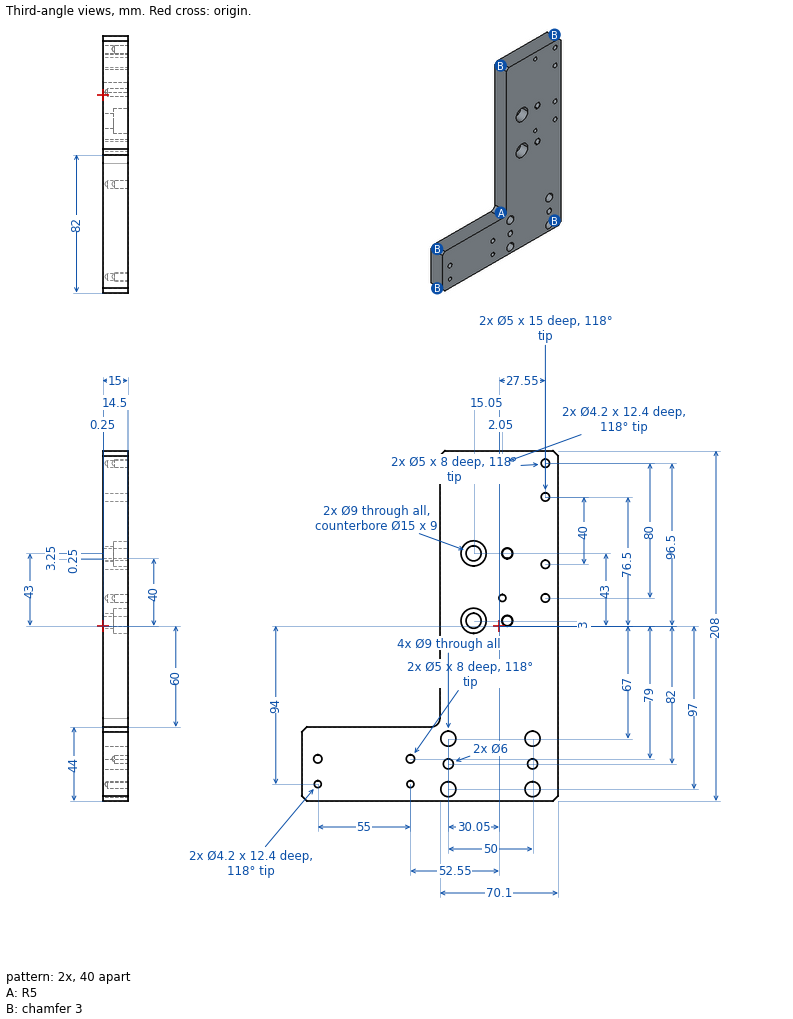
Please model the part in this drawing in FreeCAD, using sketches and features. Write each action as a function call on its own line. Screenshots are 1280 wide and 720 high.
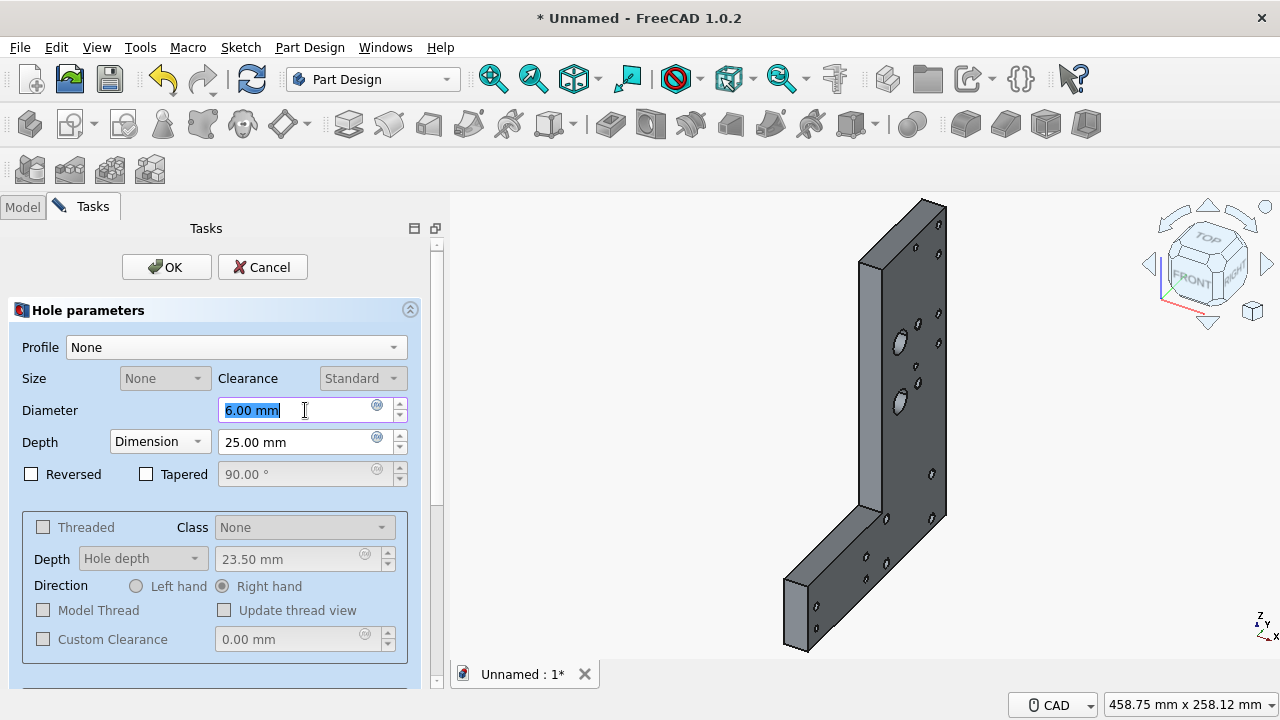
text(9)
key(Tab)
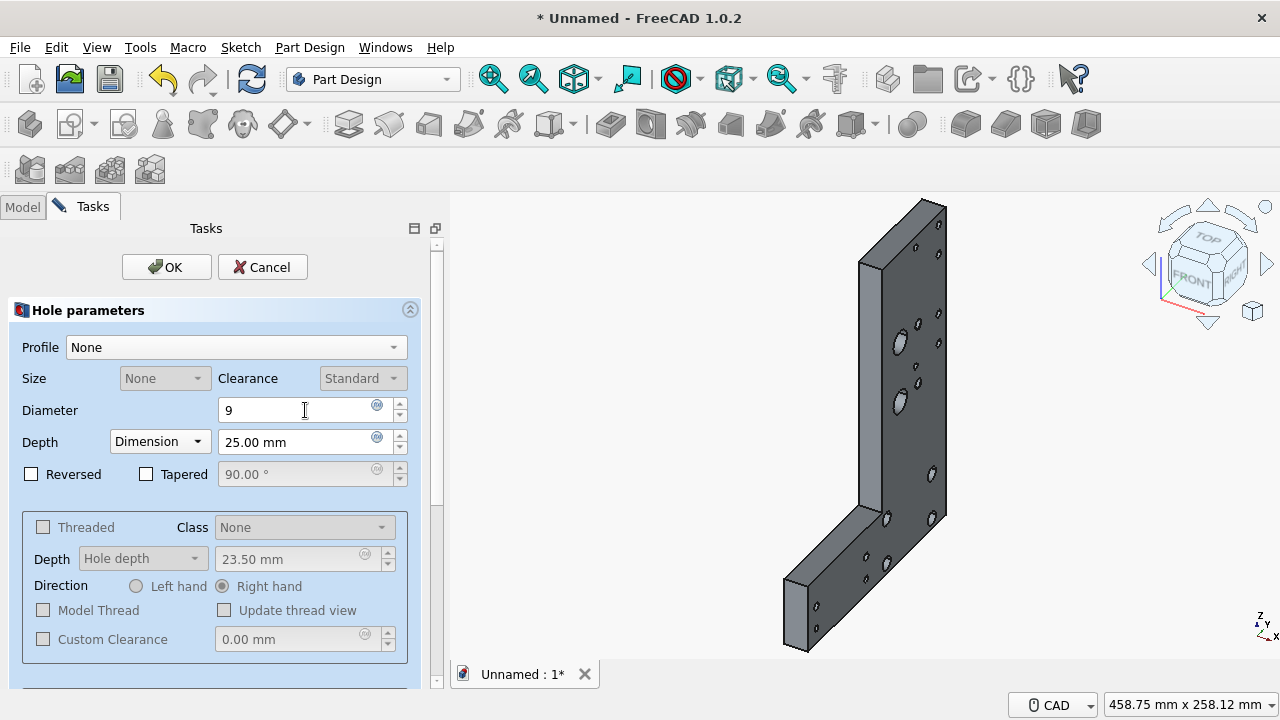
click(161, 442)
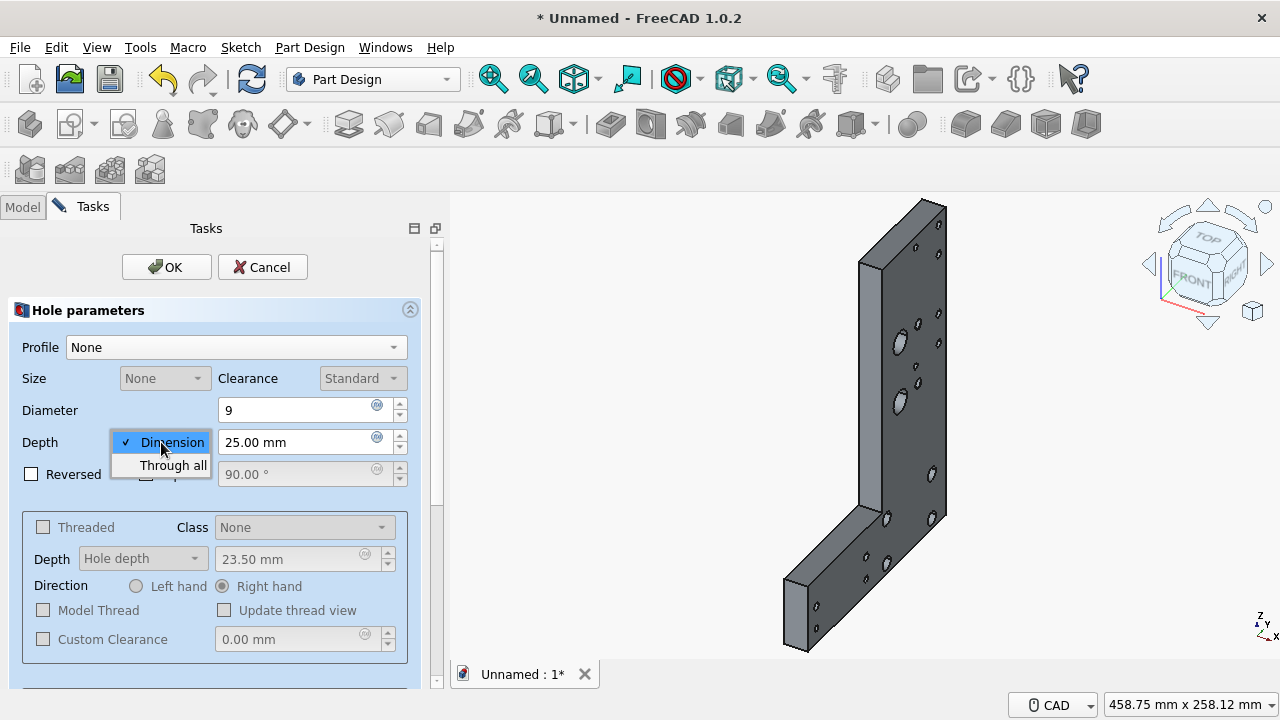
click(160, 466)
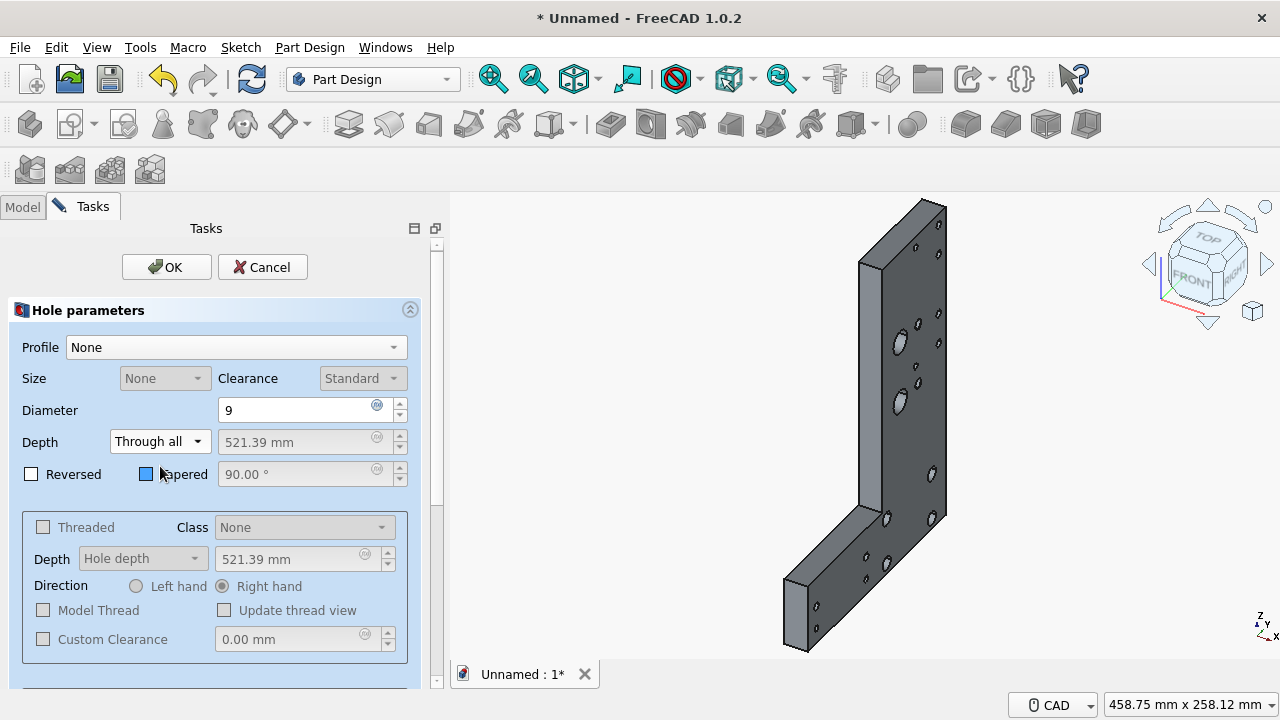
click(167, 267)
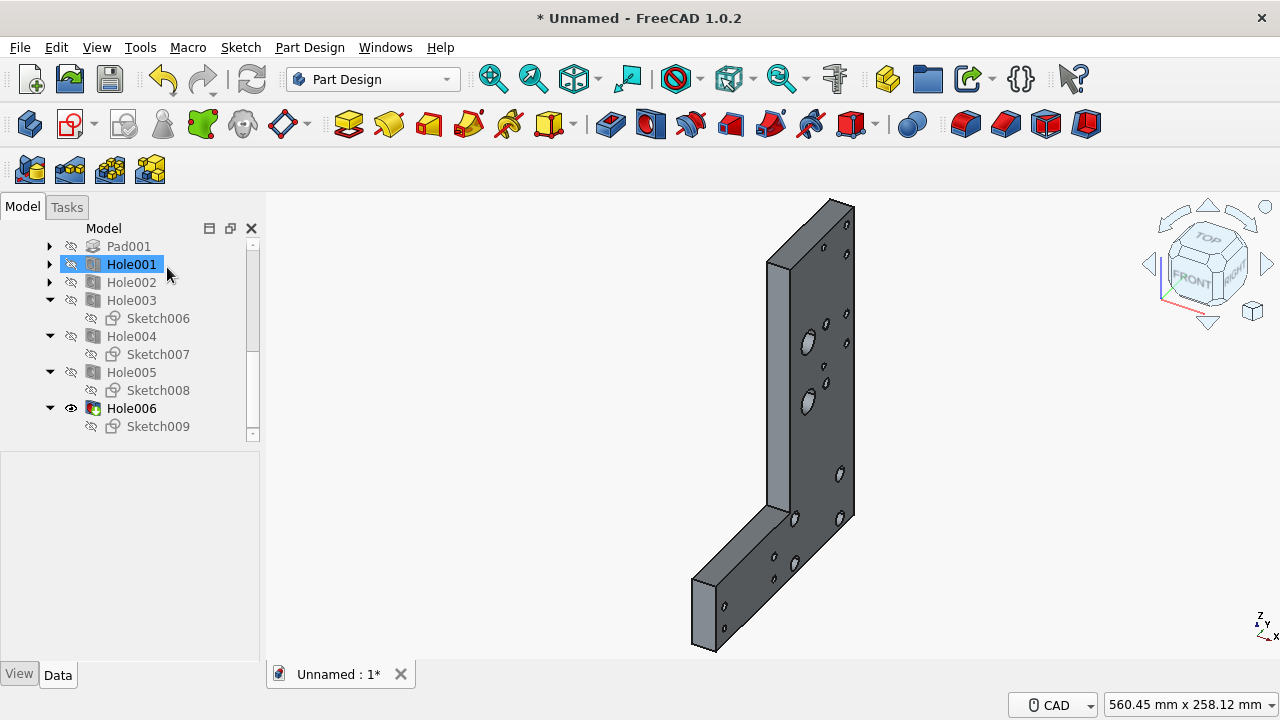
click(824, 433)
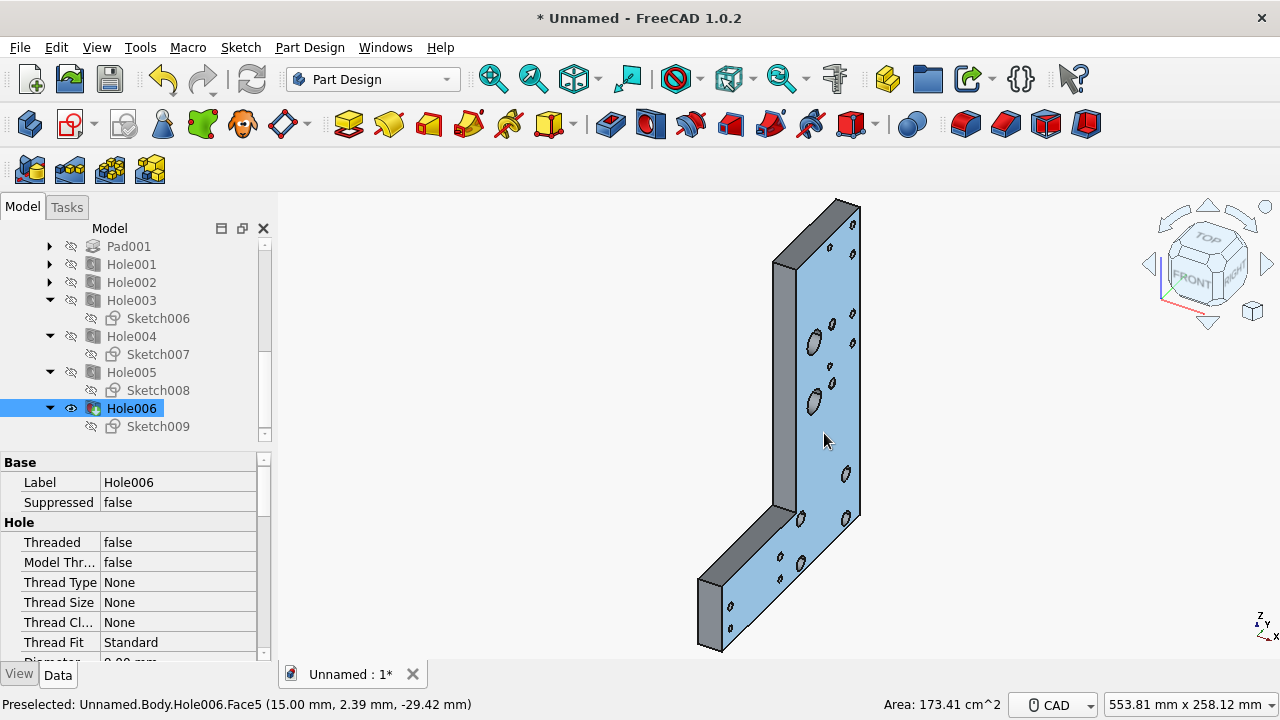
click(70, 124)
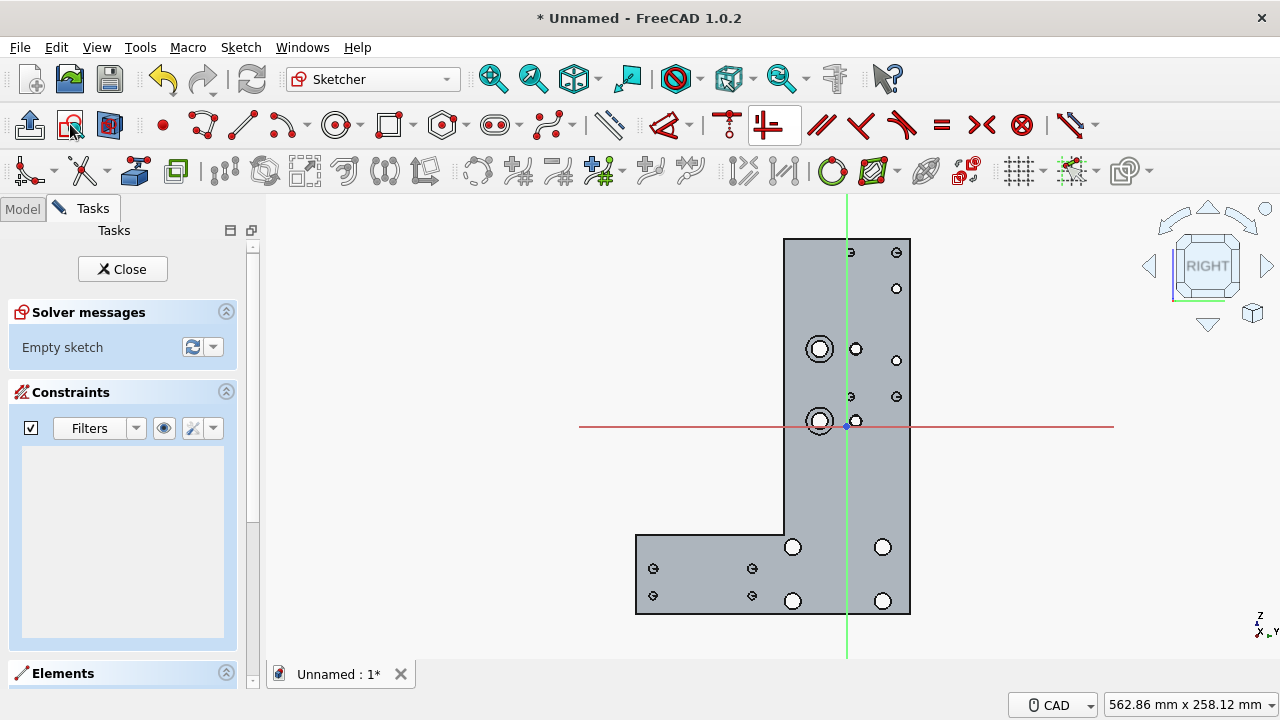
scroll(1000, 596, up, 3)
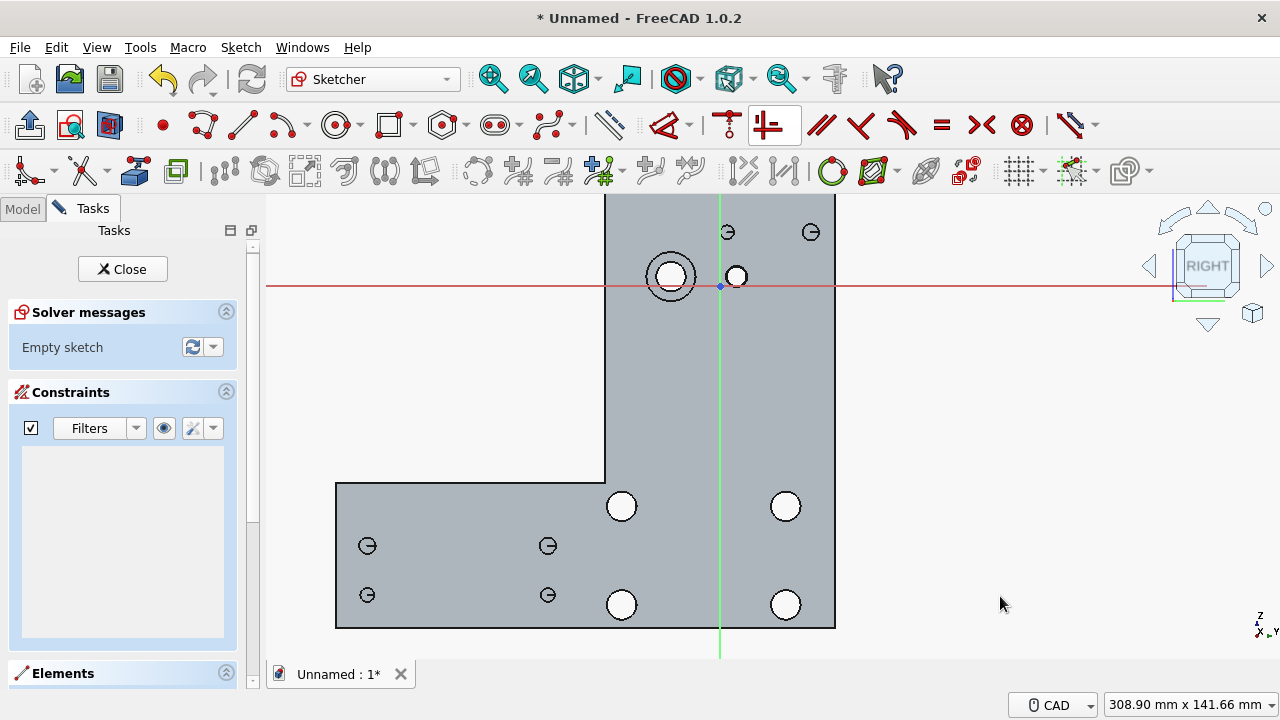
click(336, 126)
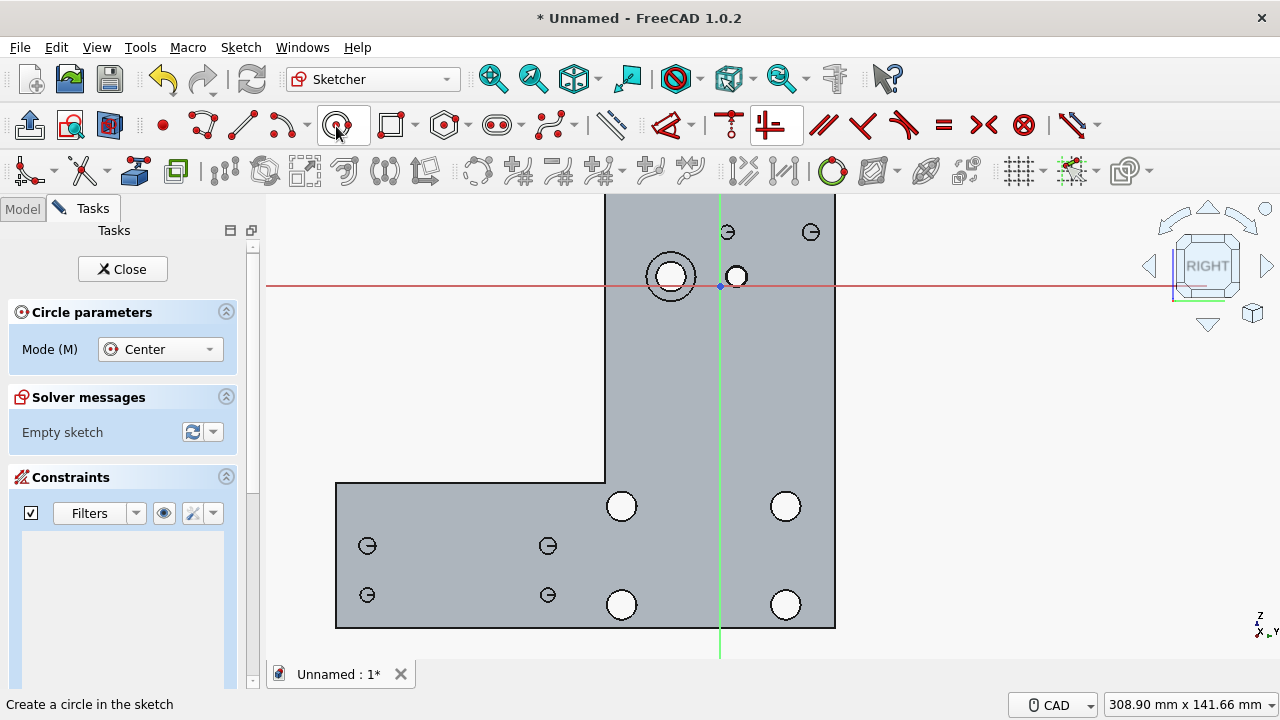
scroll(622, 556, up, 5)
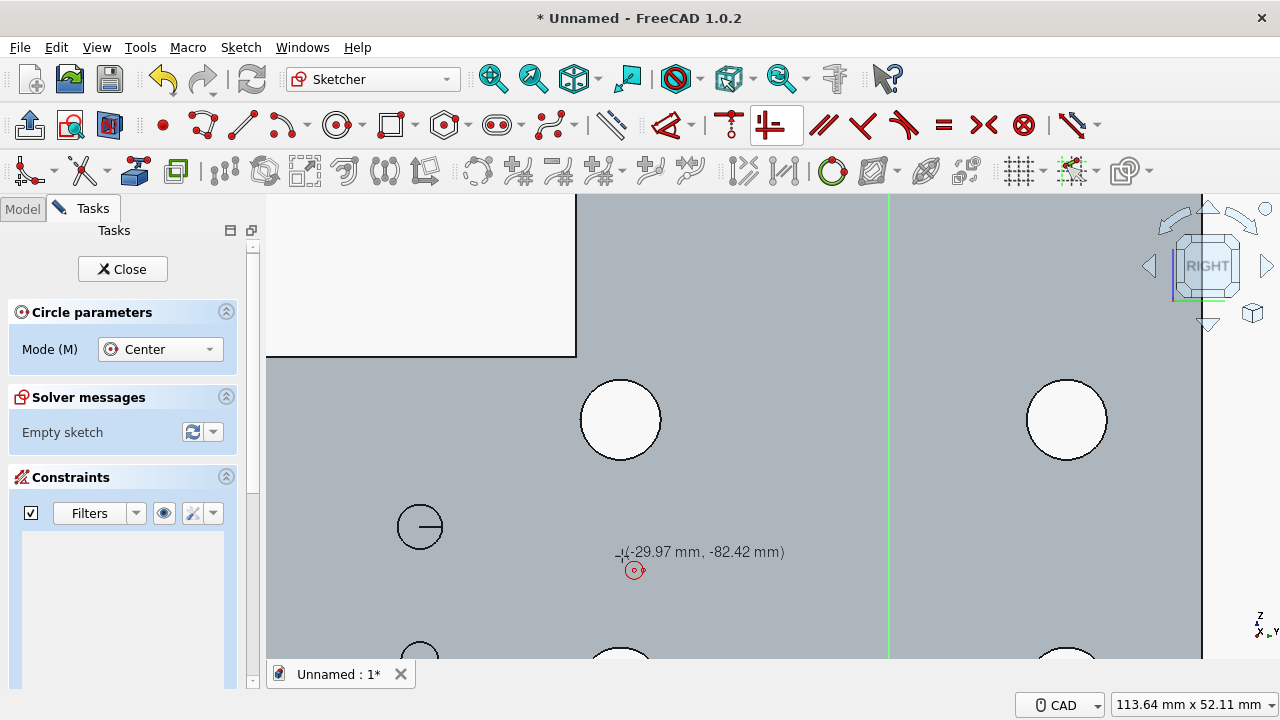
click(621, 554)
click(640, 535)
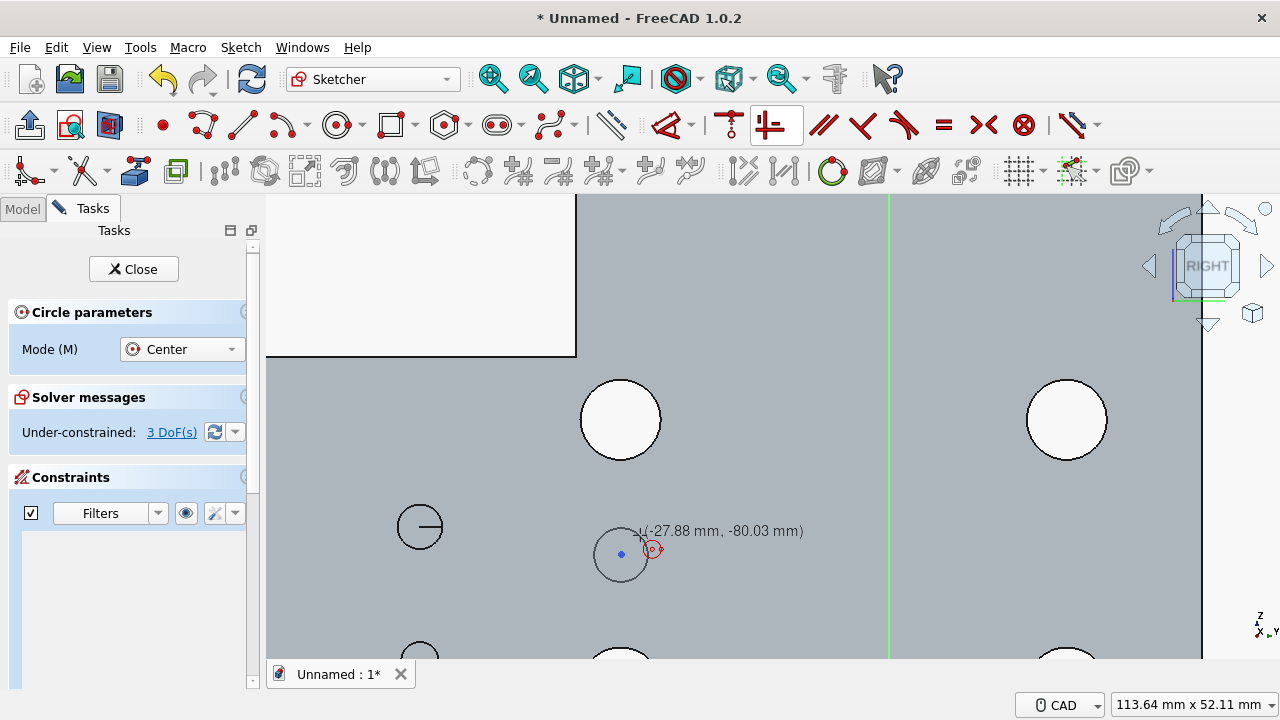
click(1067, 554)
click(1086, 535)
key(Escape)